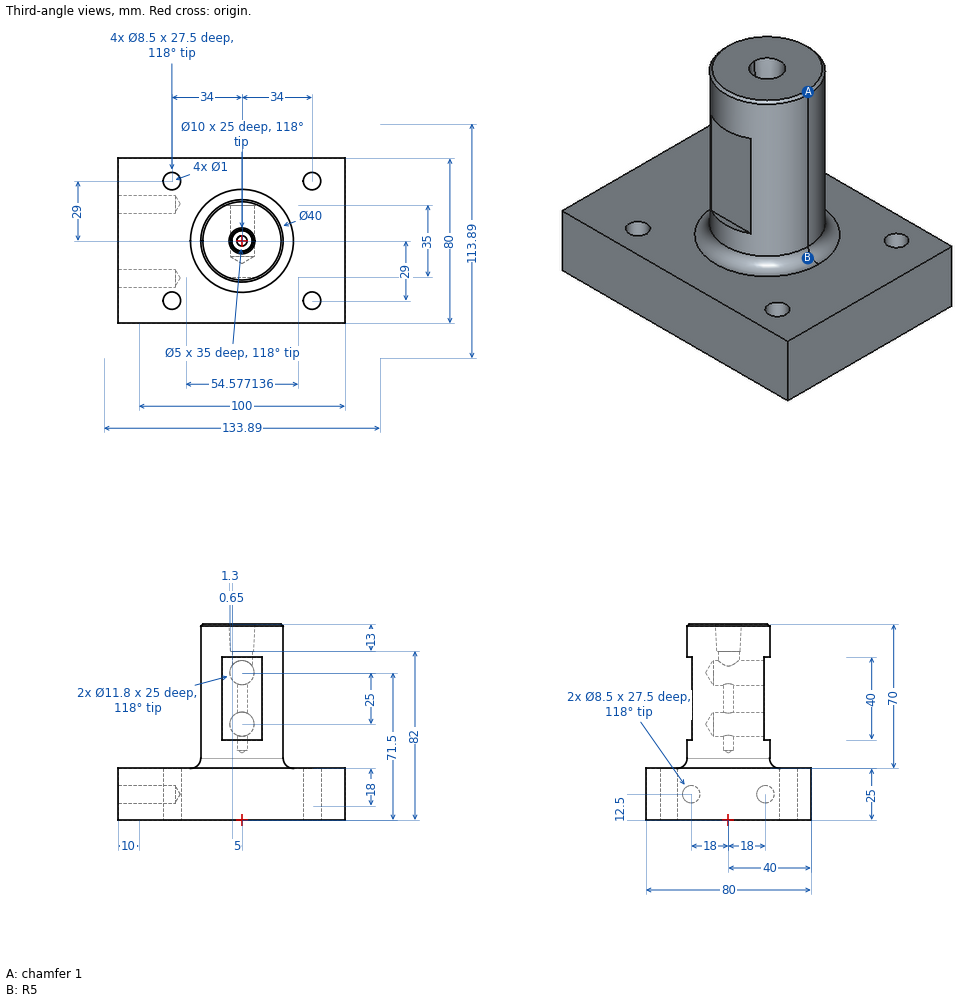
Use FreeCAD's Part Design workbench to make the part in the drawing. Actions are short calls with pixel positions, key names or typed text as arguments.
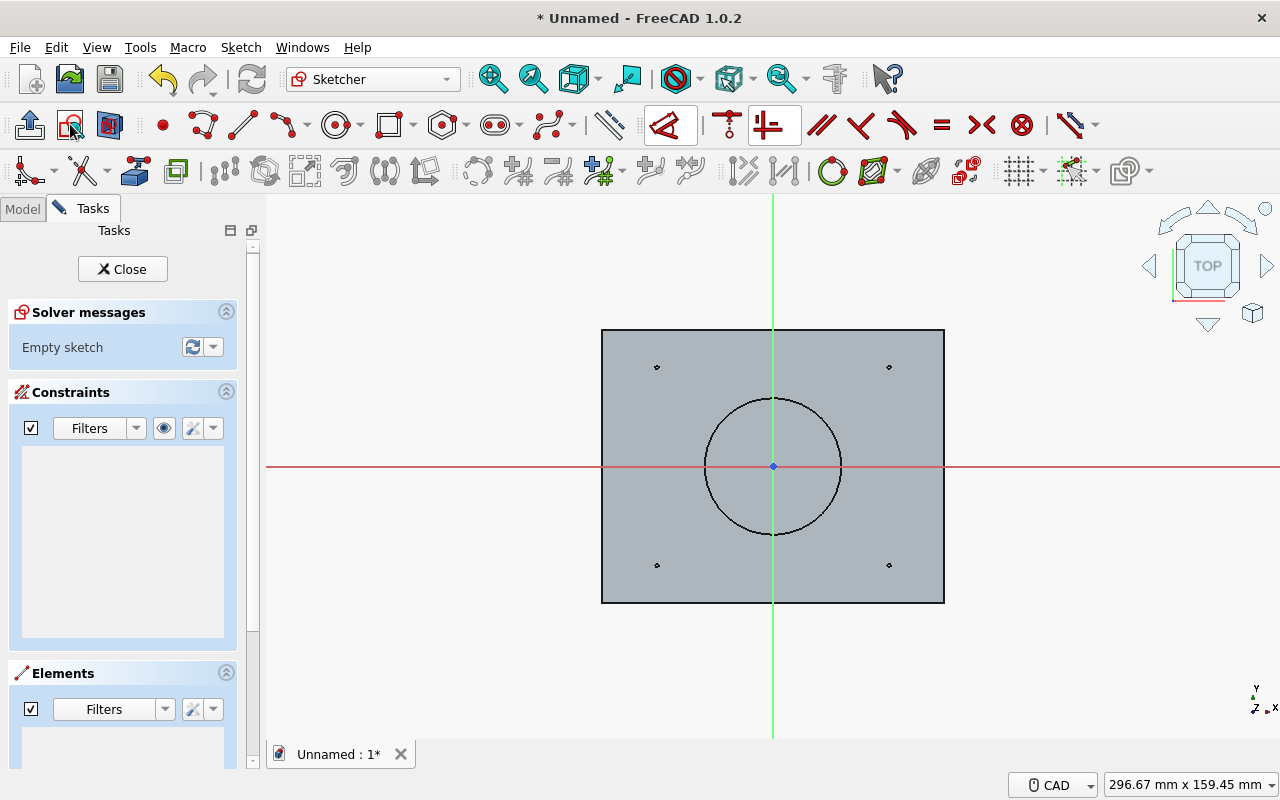
scroll(780, 466, up, 12)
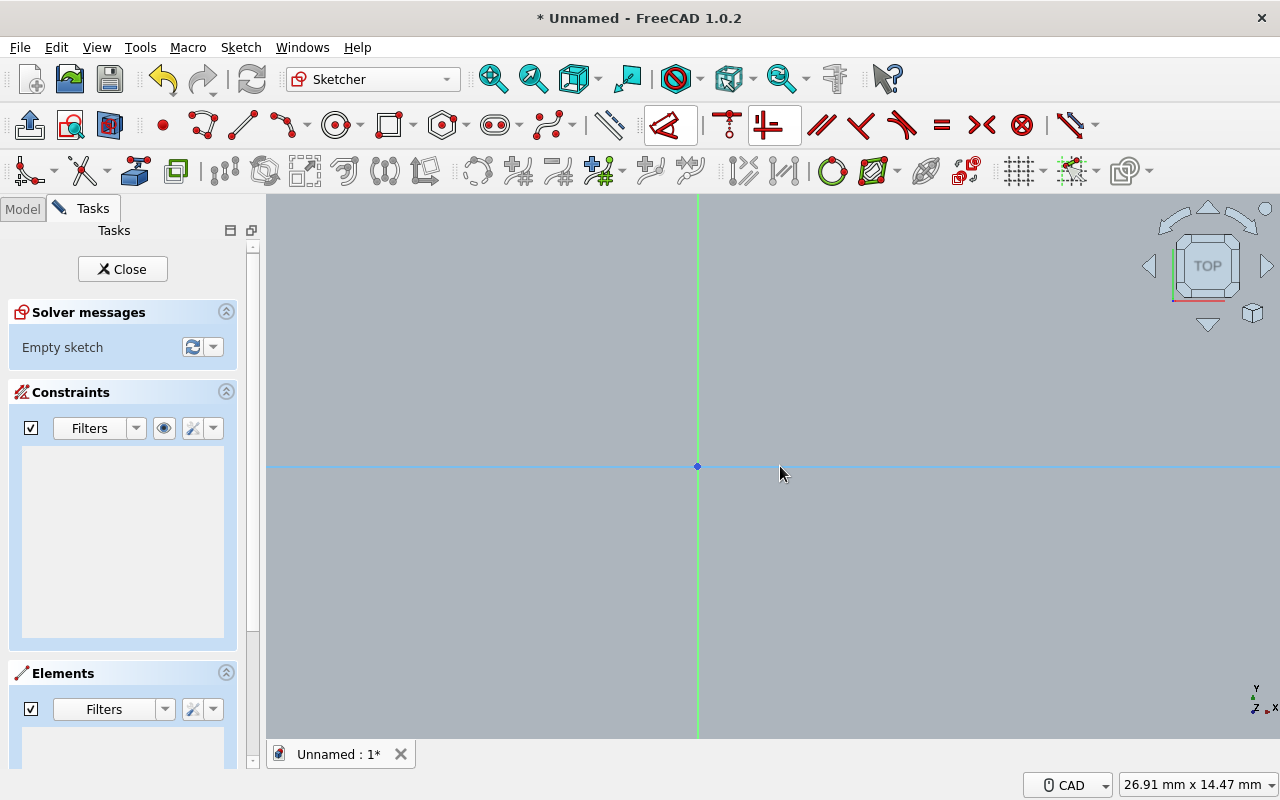
click(336, 126)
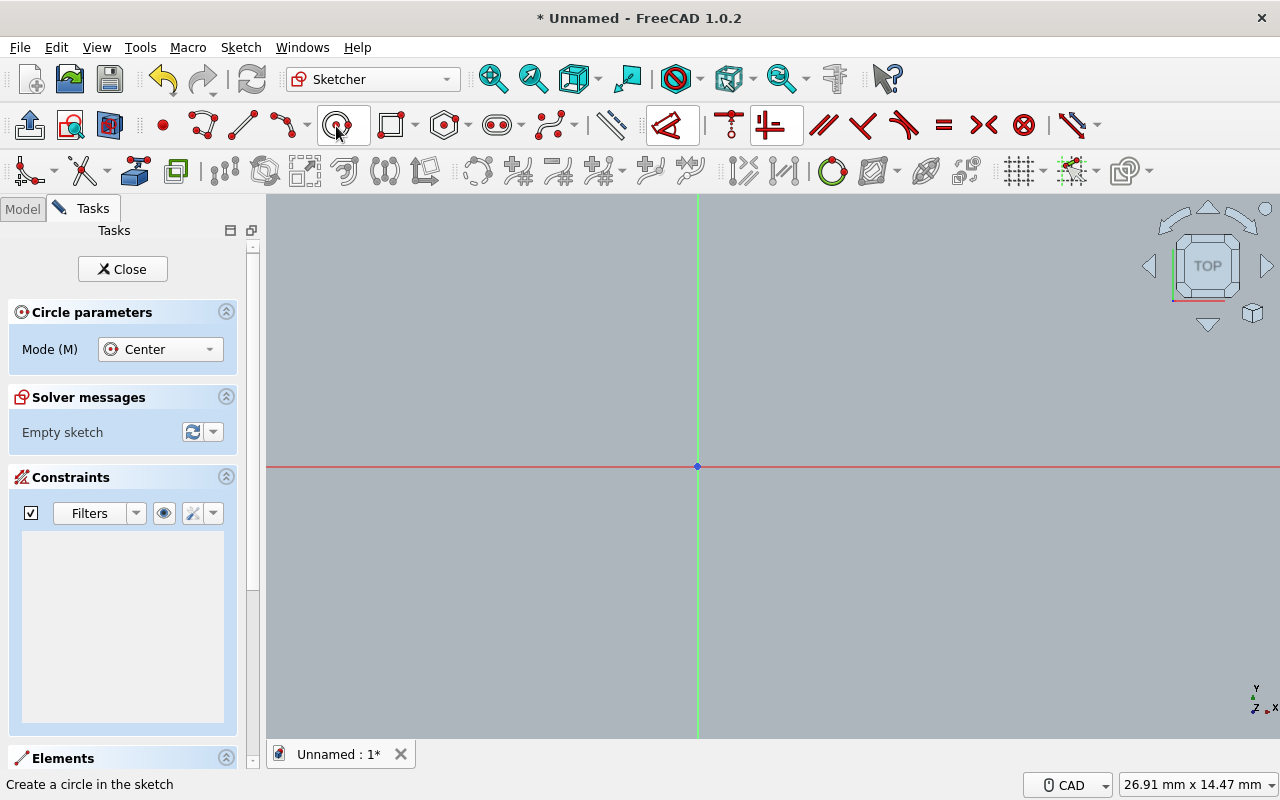
click(698, 466)
click(831, 333)
key(Escape)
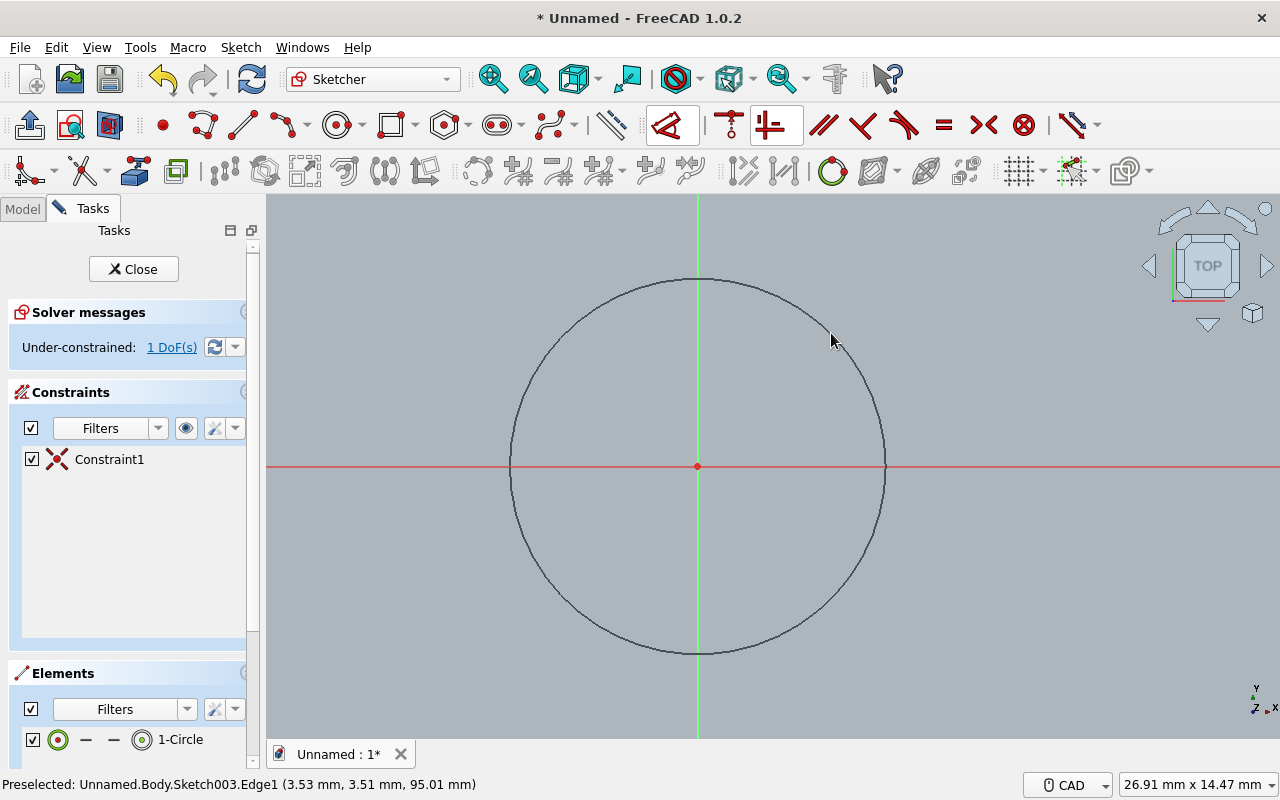
click(830, 333)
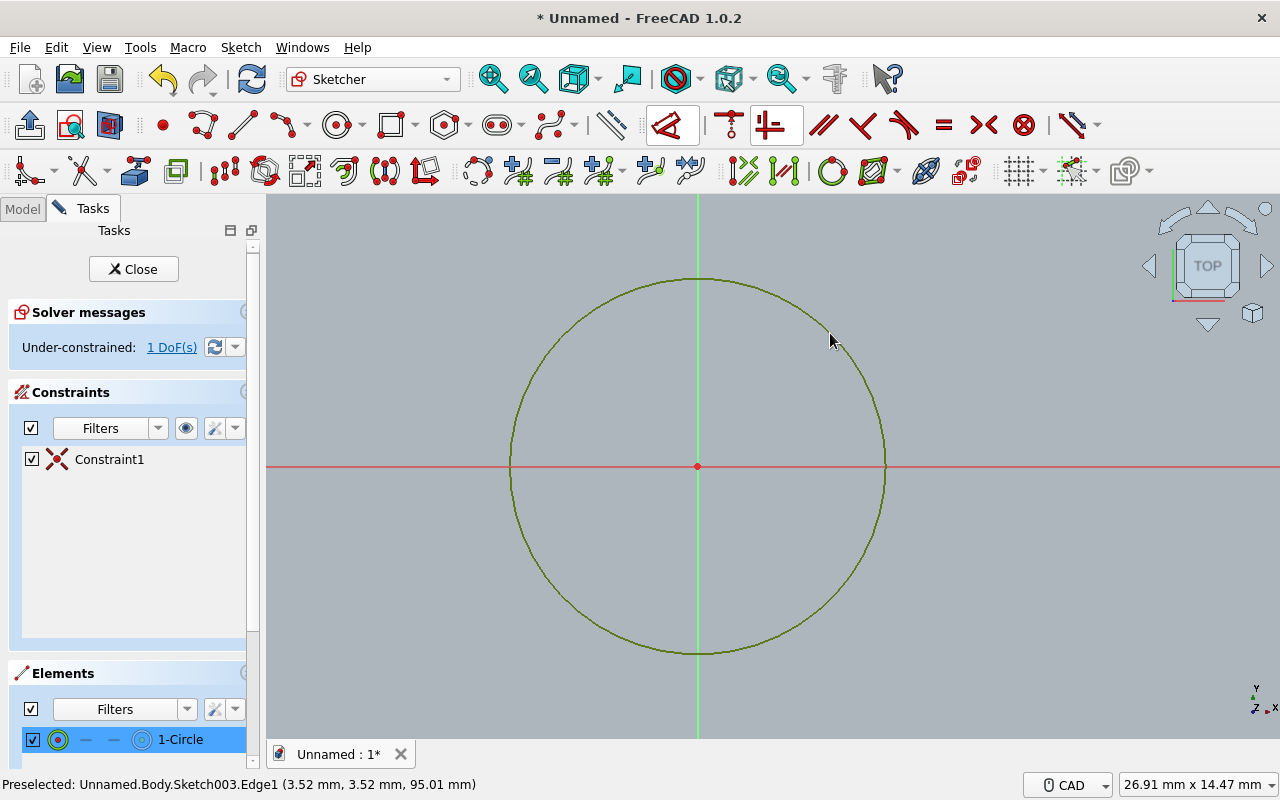
key(k)
key(o)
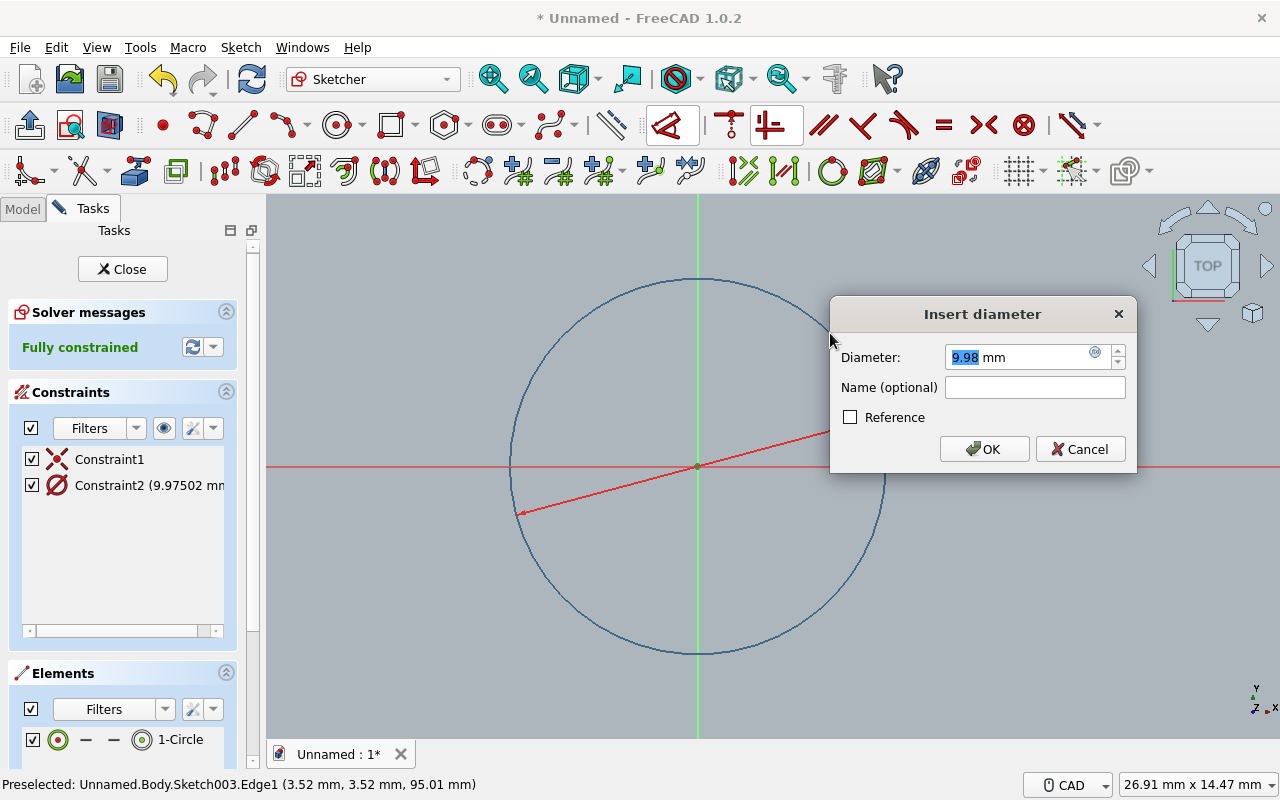
text(10)
key(Return)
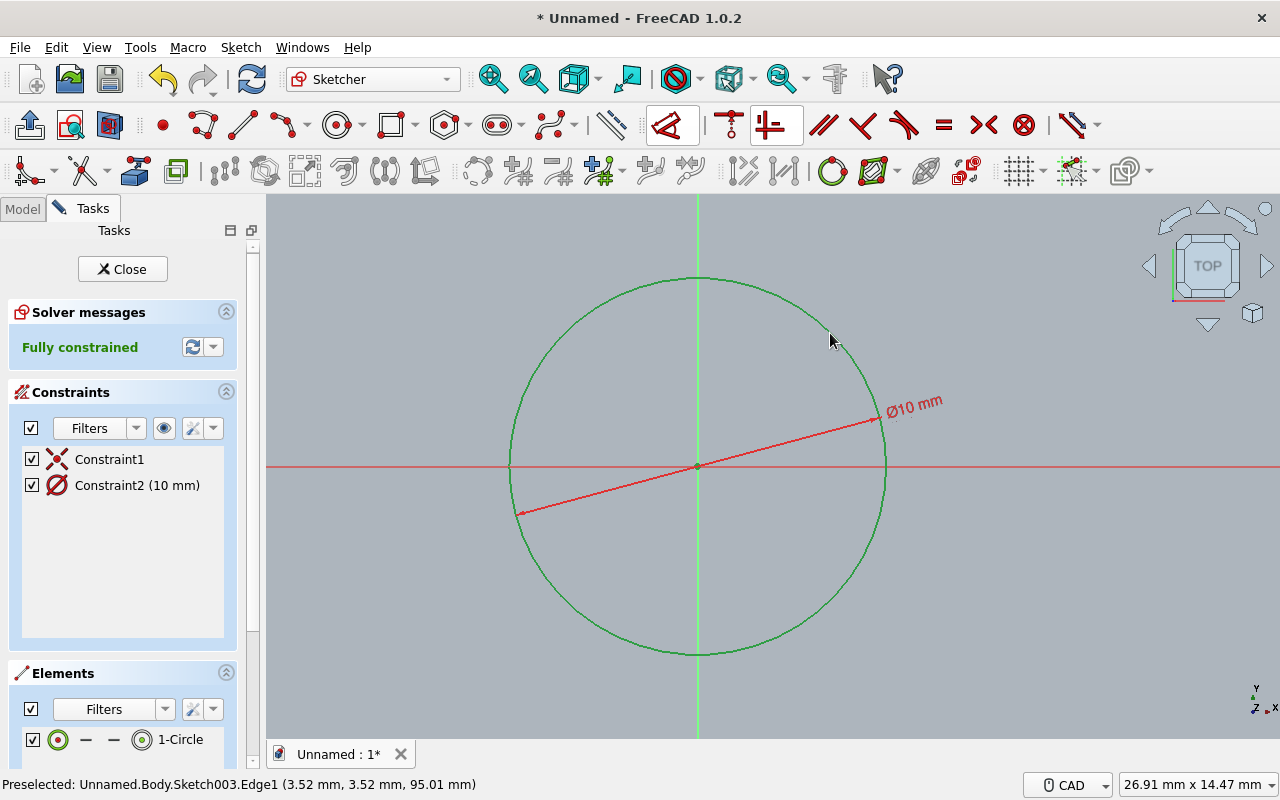
click(123, 269)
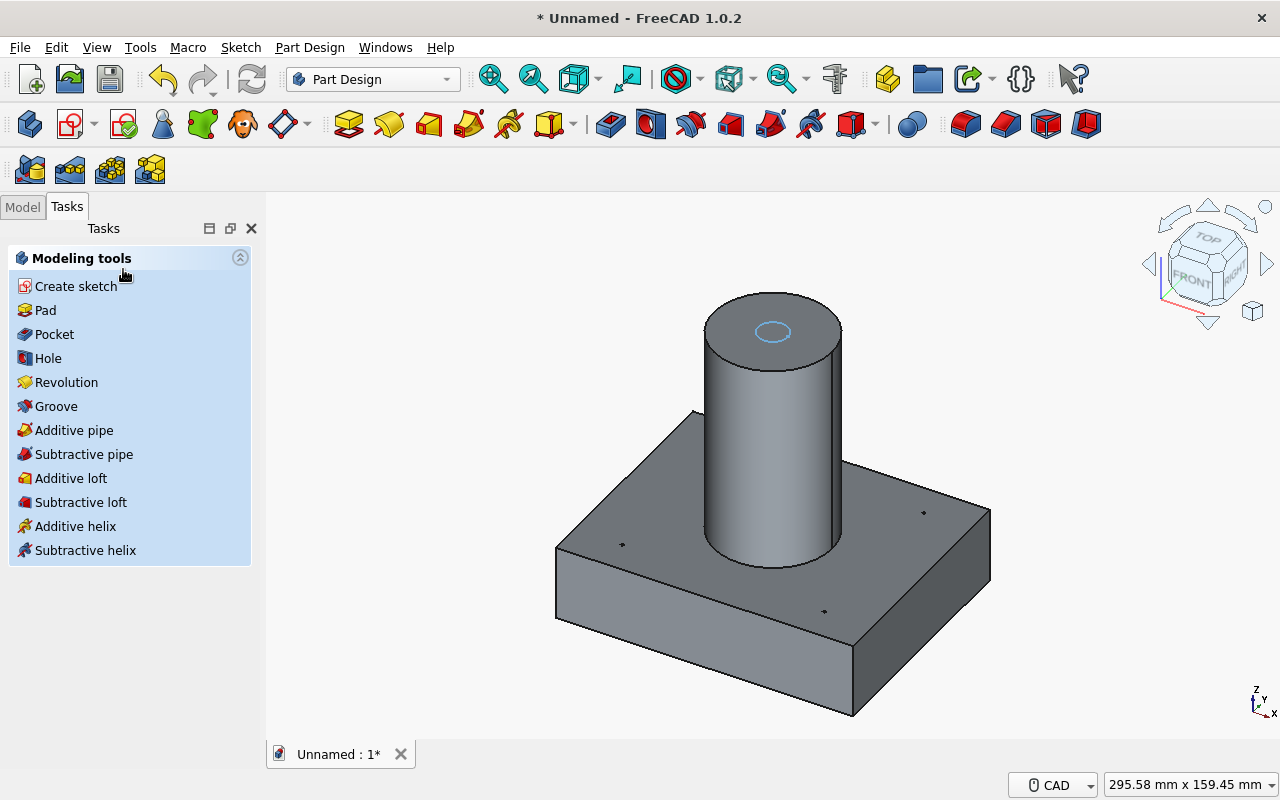
click(652, 124)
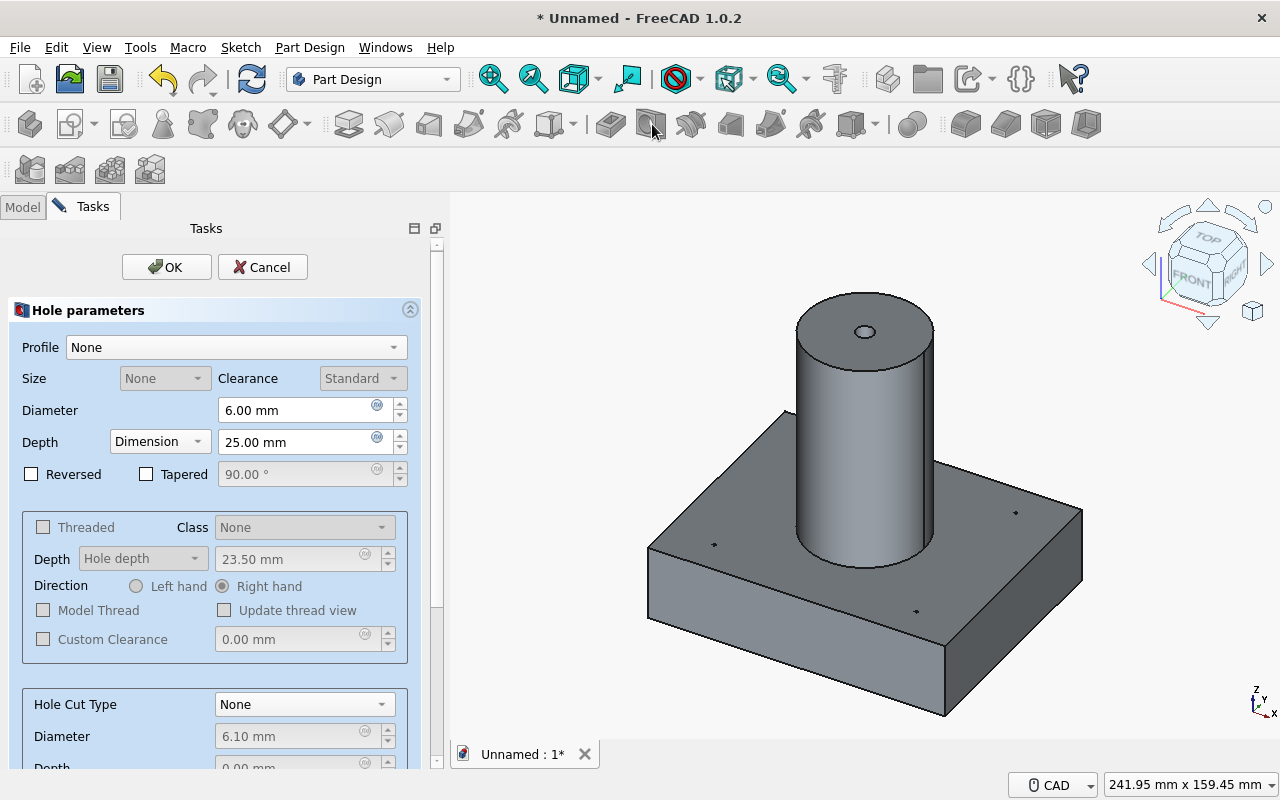
triple_click(305, 410)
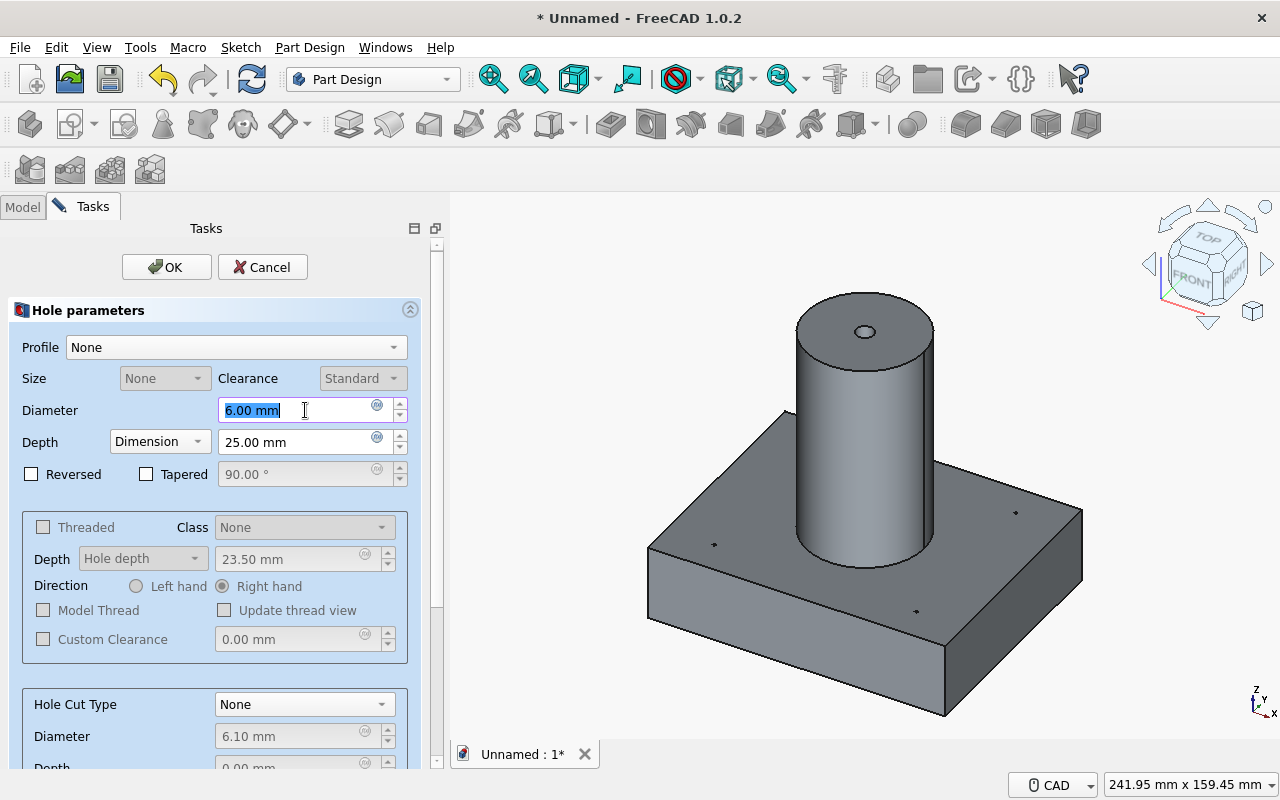
text(10)
key(Tab)